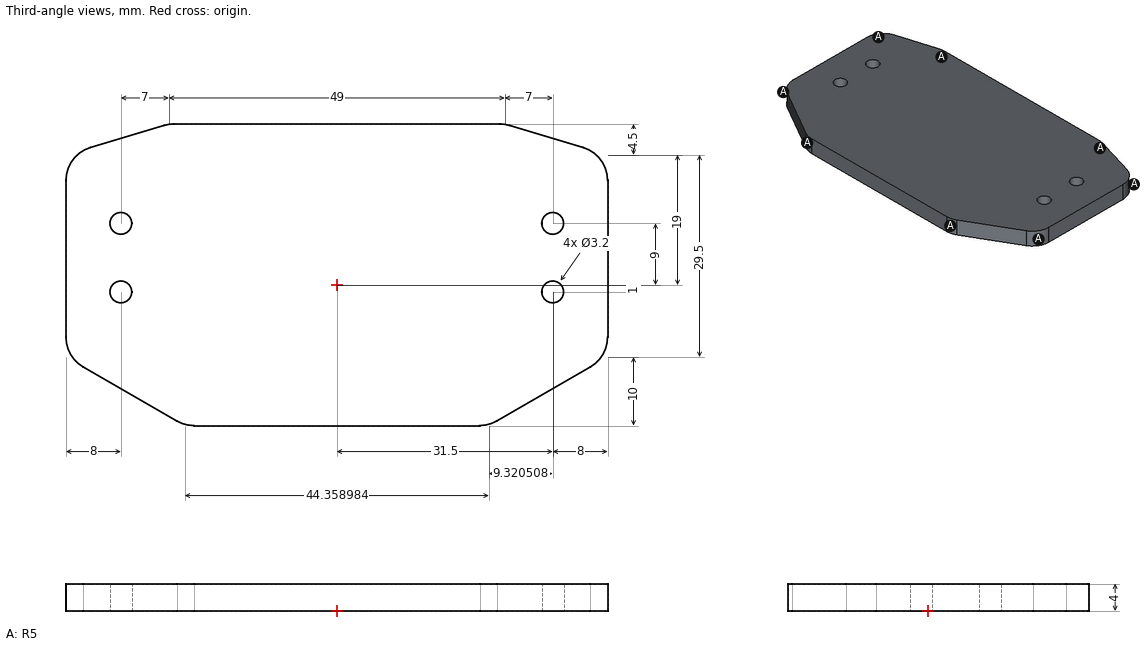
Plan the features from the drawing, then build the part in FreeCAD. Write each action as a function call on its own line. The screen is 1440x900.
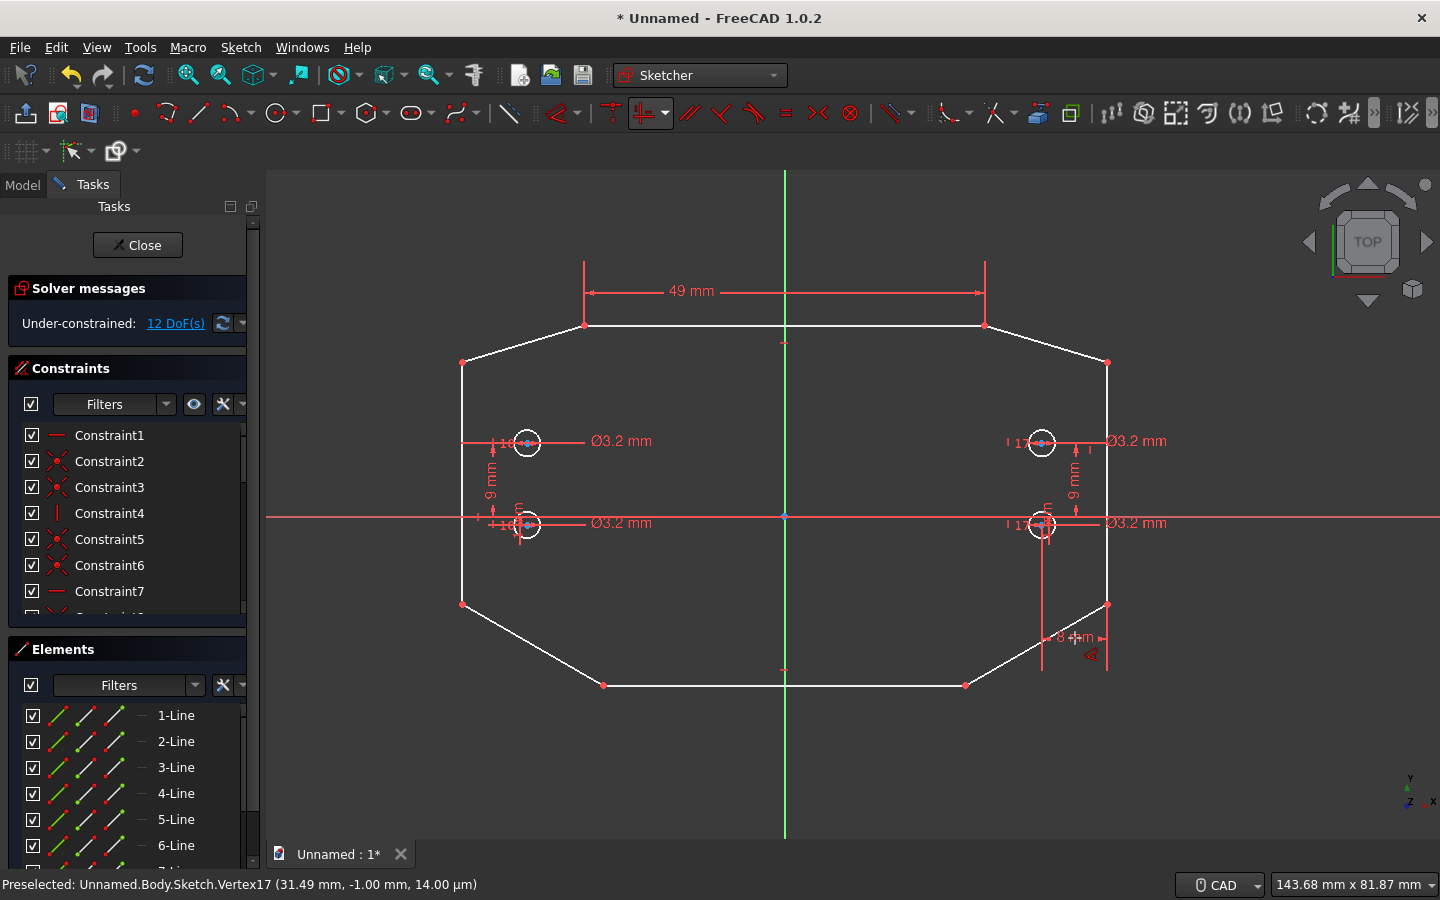
click(462, 604)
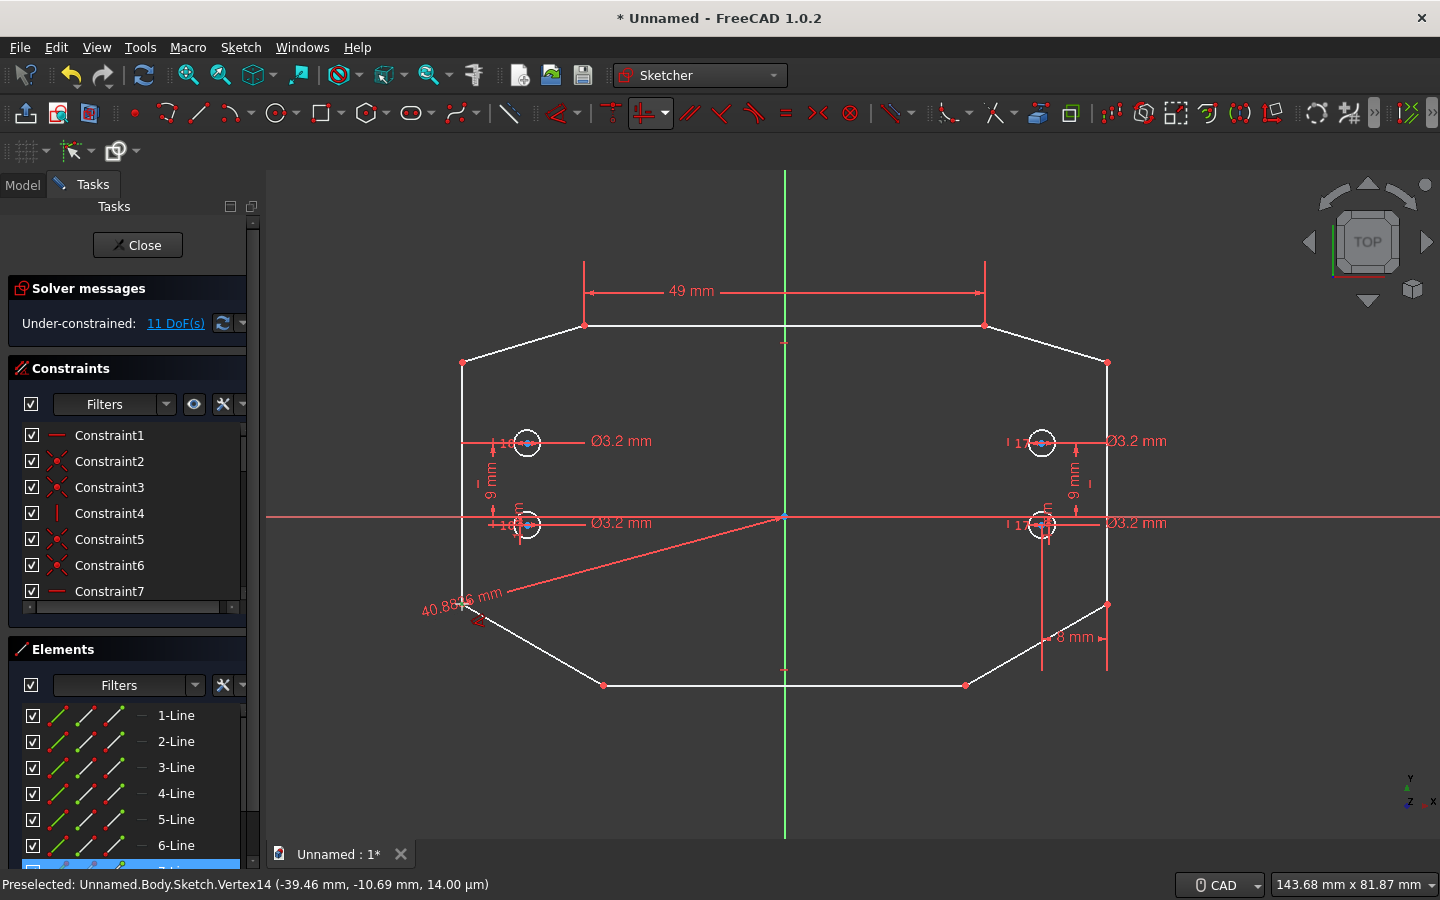
click(527, 525)
click(495, 638)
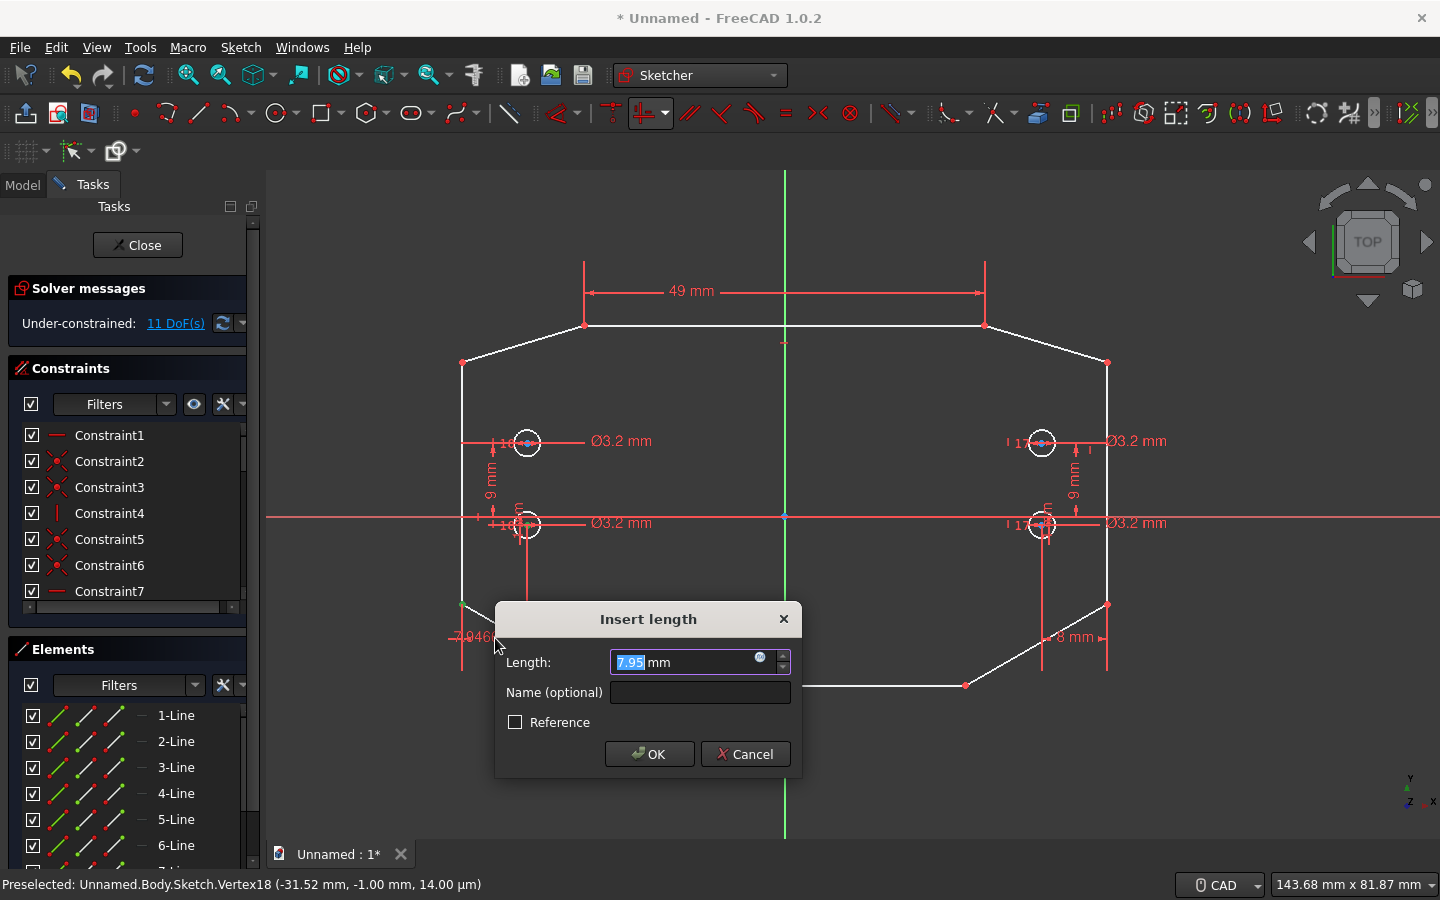
text(8)
key(Return)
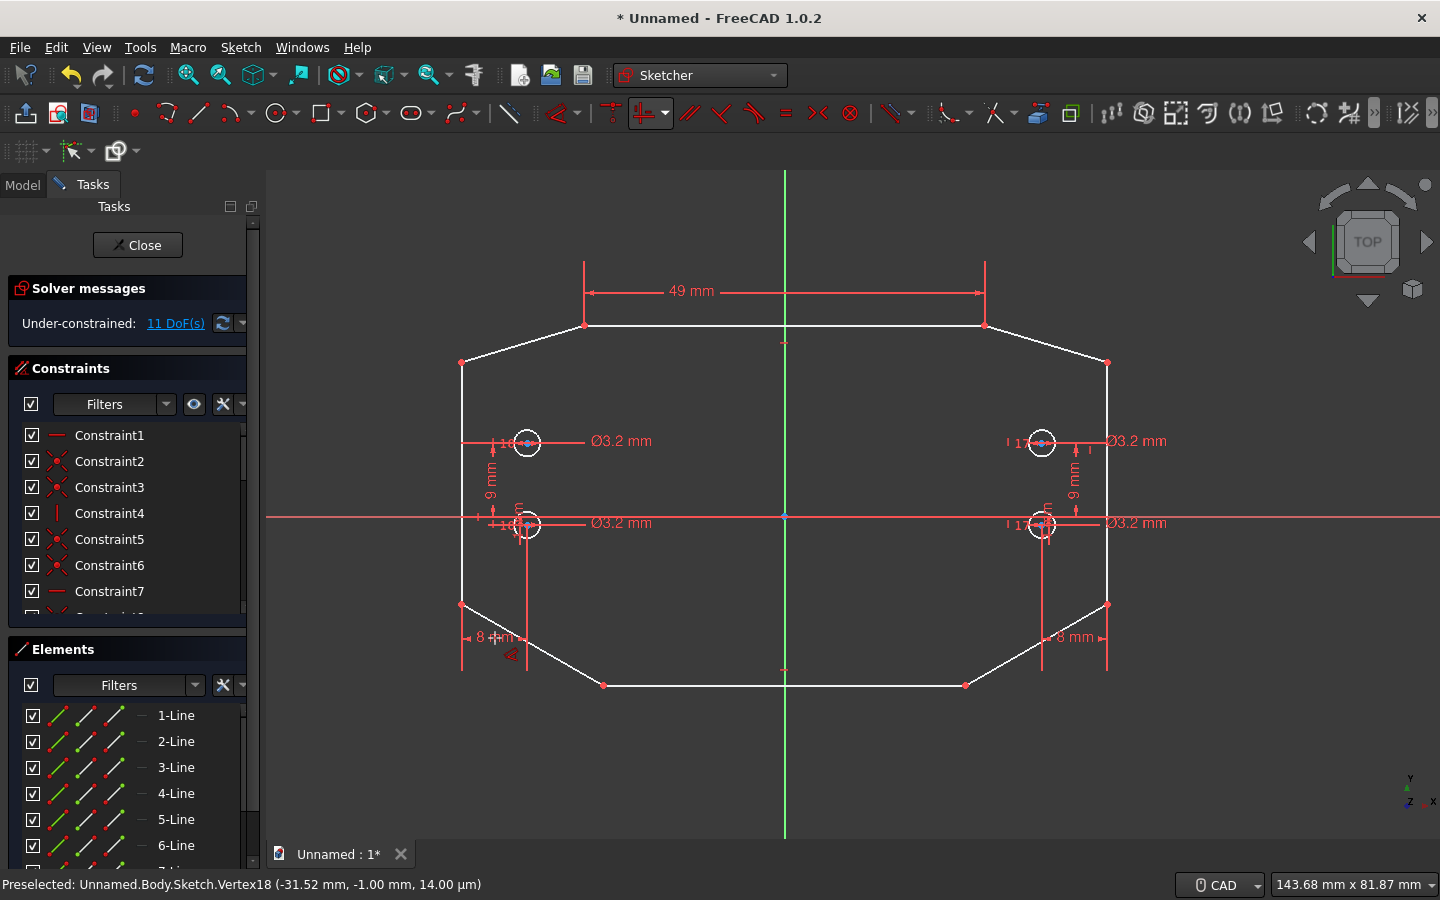
click(985, 326)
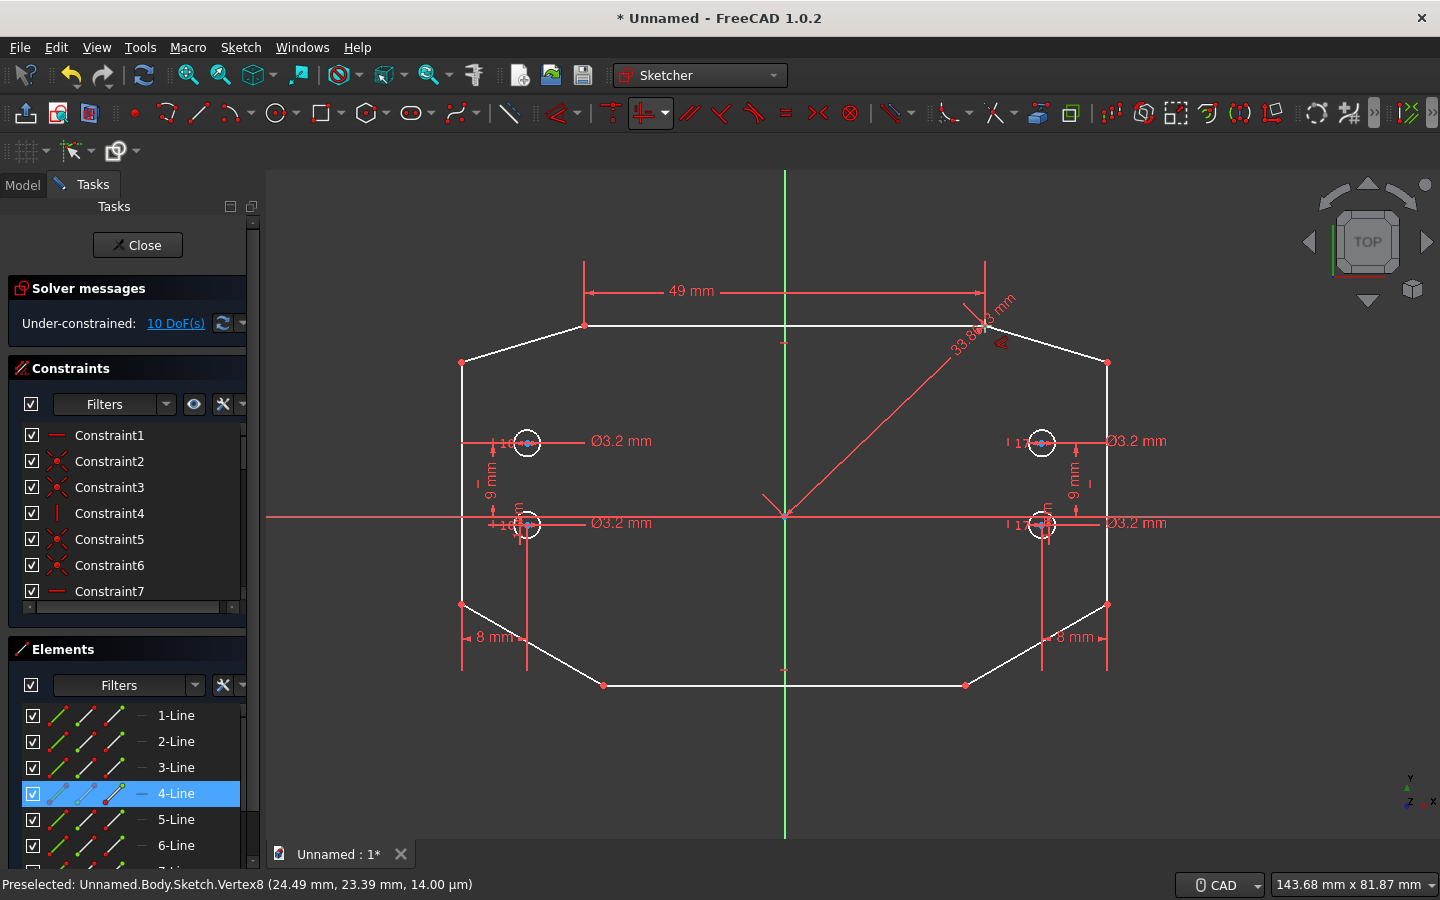
click(1042, 443)
click(1013, 292)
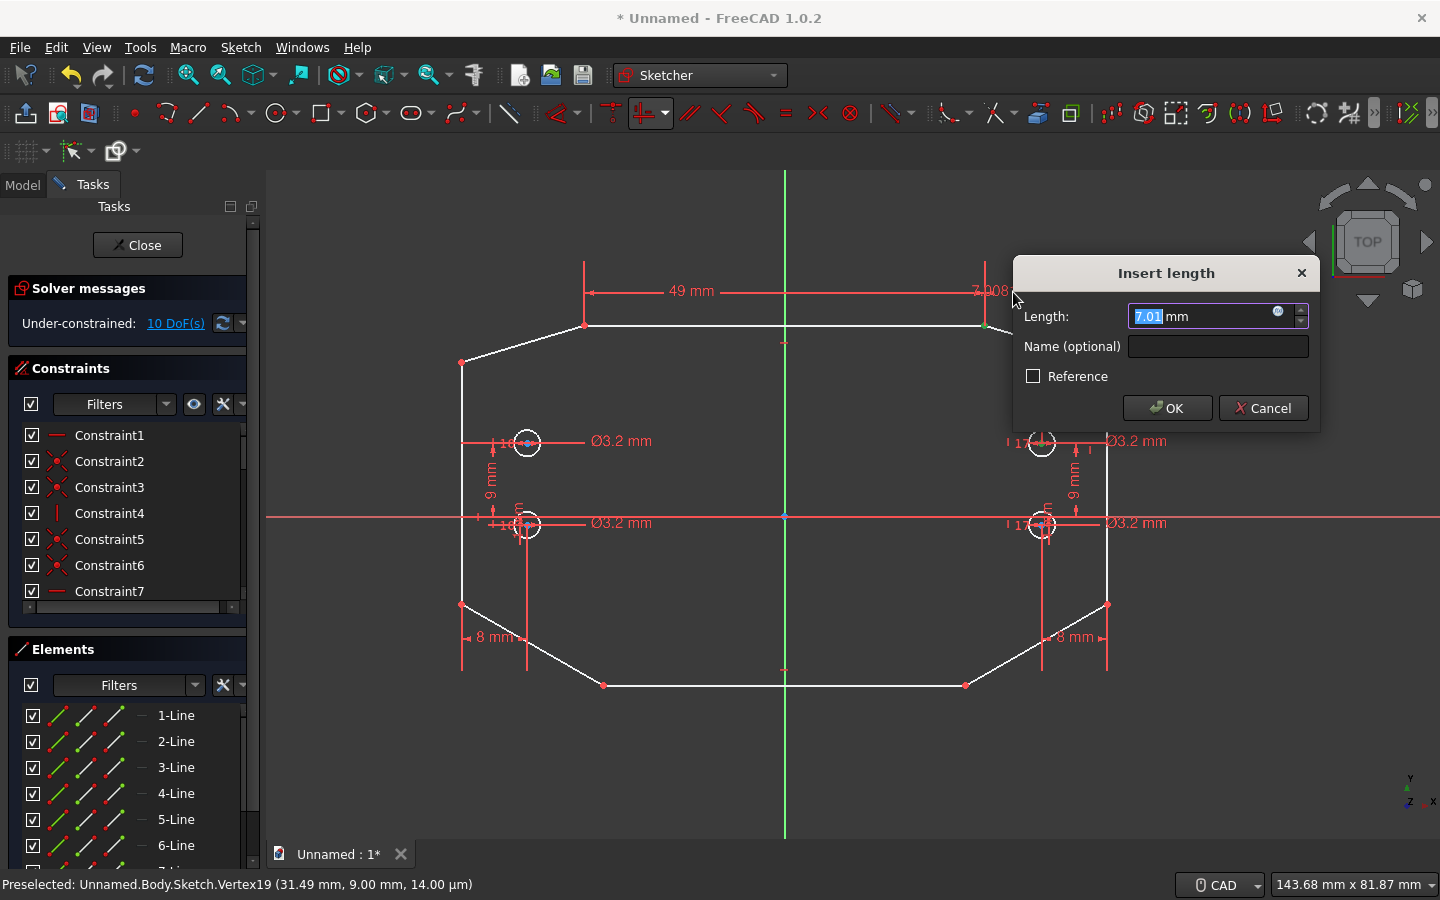
text(7)
key(Return)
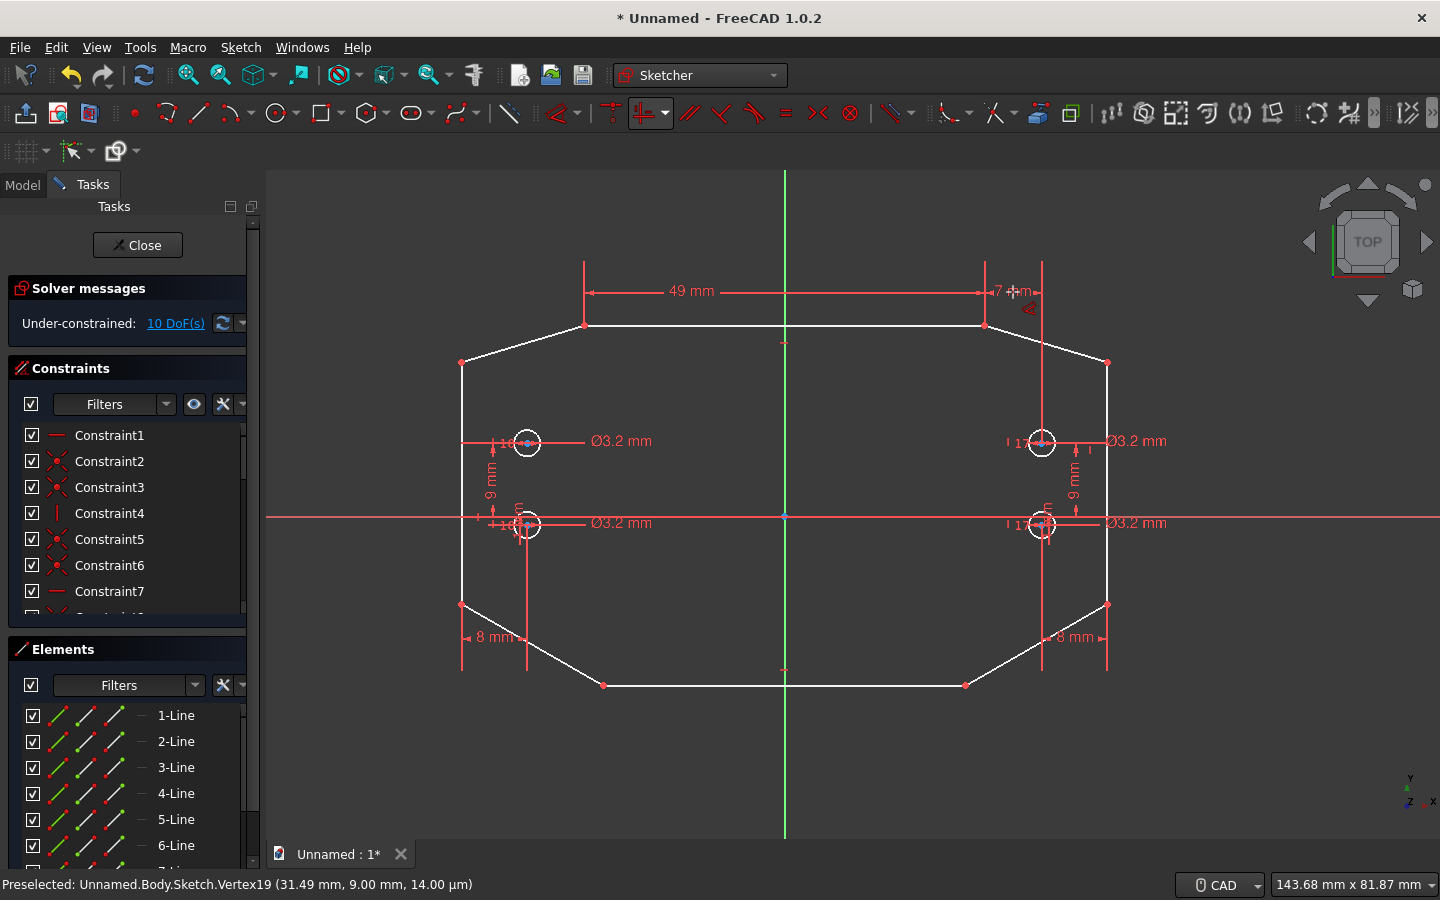
click(584, 326)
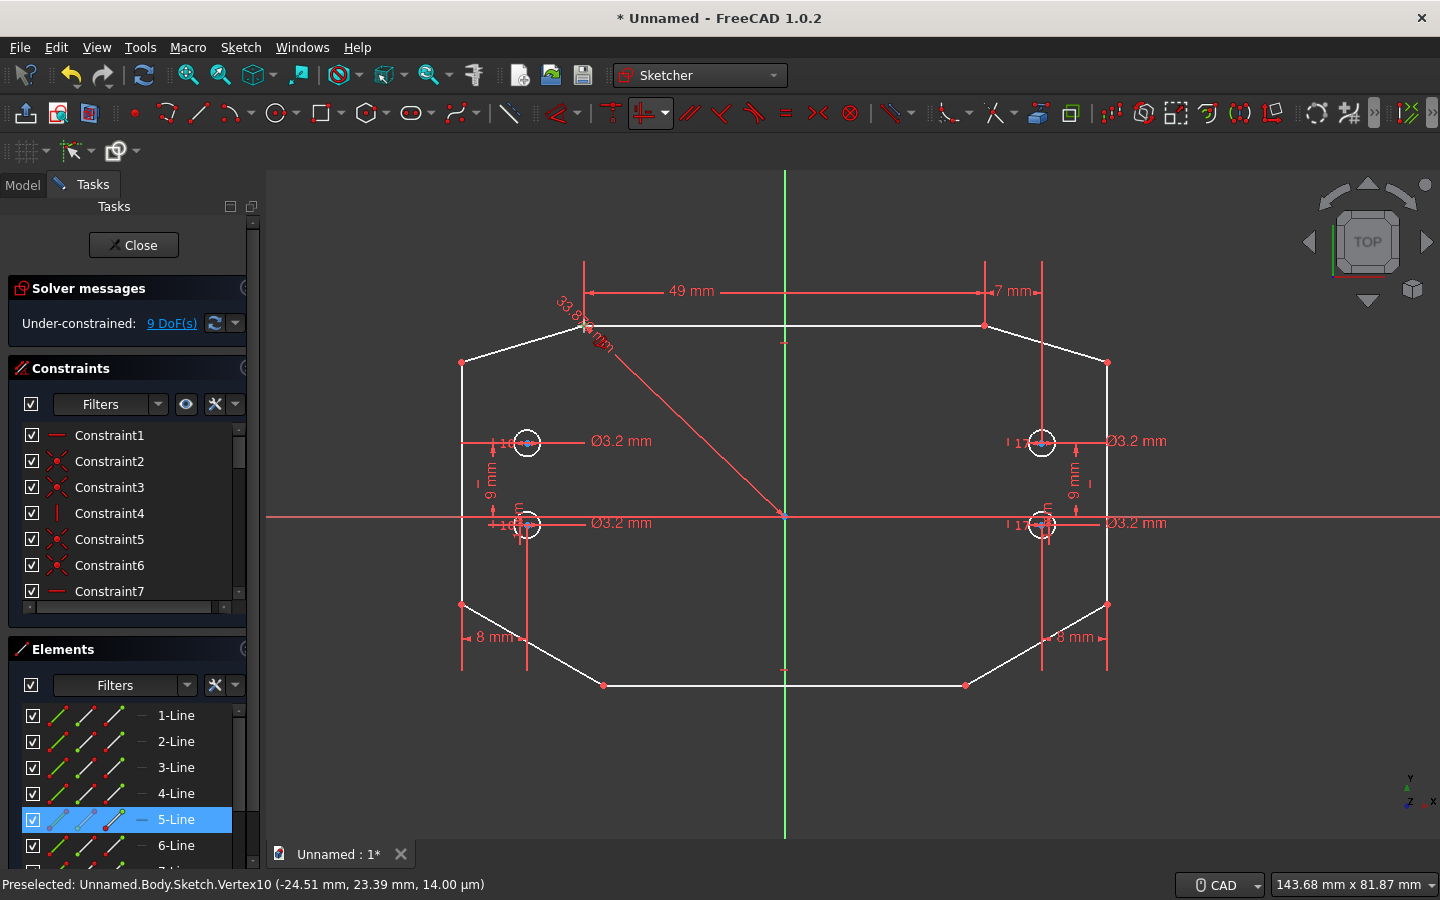
click(527, 443)
click(556, 292)